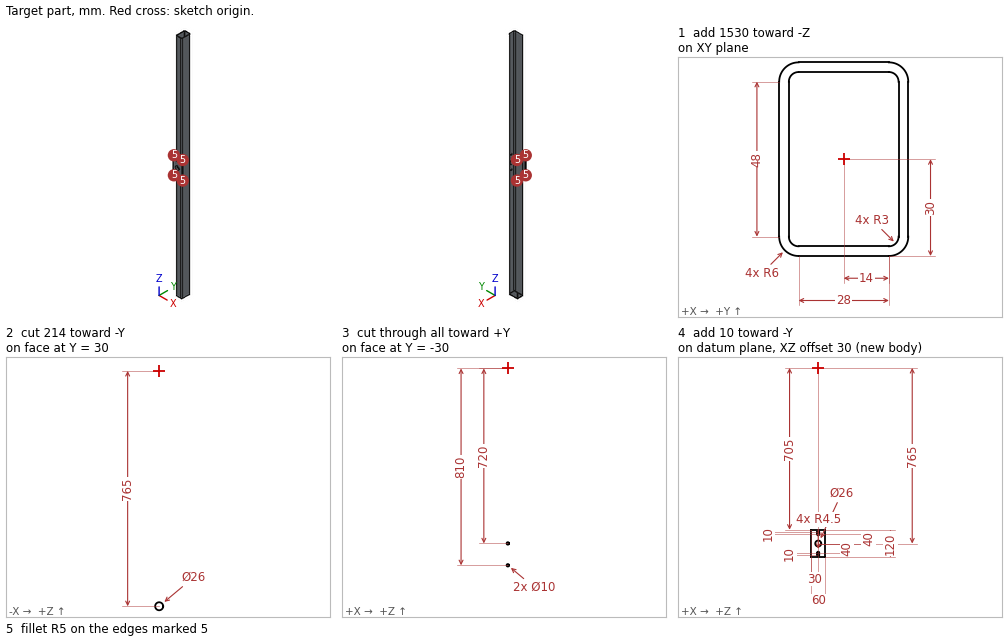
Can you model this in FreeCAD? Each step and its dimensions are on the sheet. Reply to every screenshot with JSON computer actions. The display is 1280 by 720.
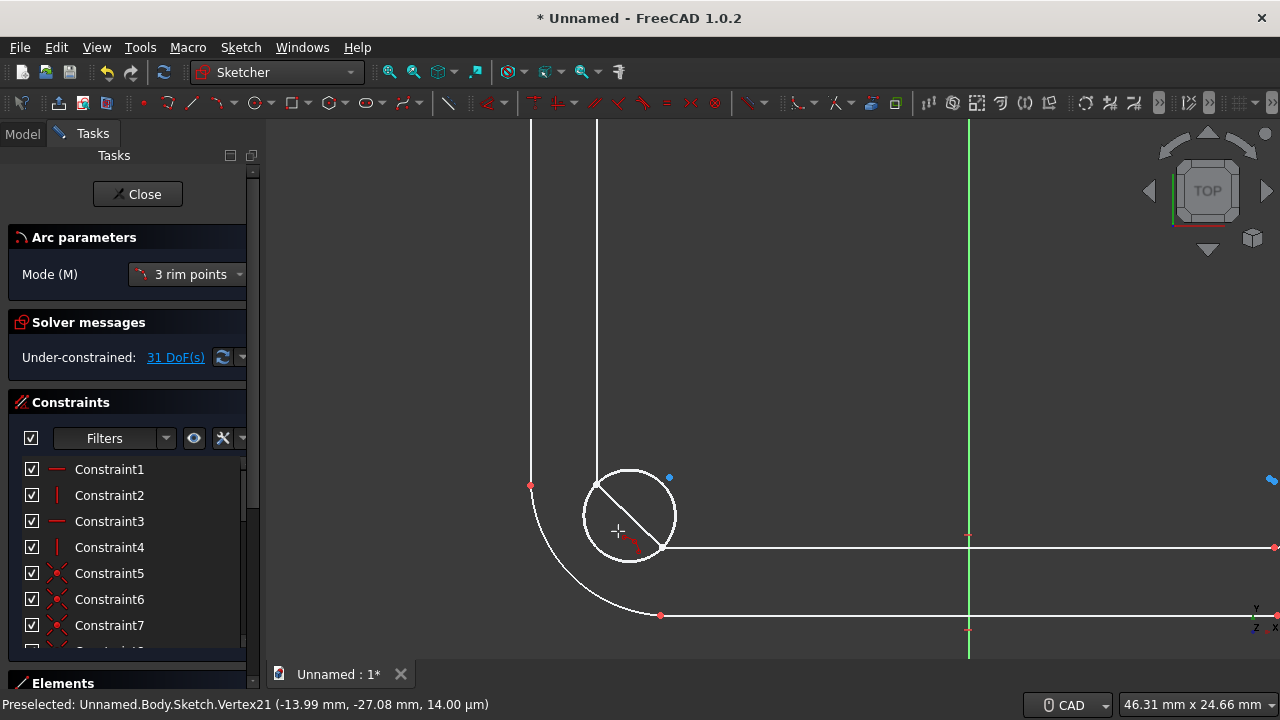
{"action": "left_click", "coordinate": [616, 527]}
{"action": "key", "text": "Escape"}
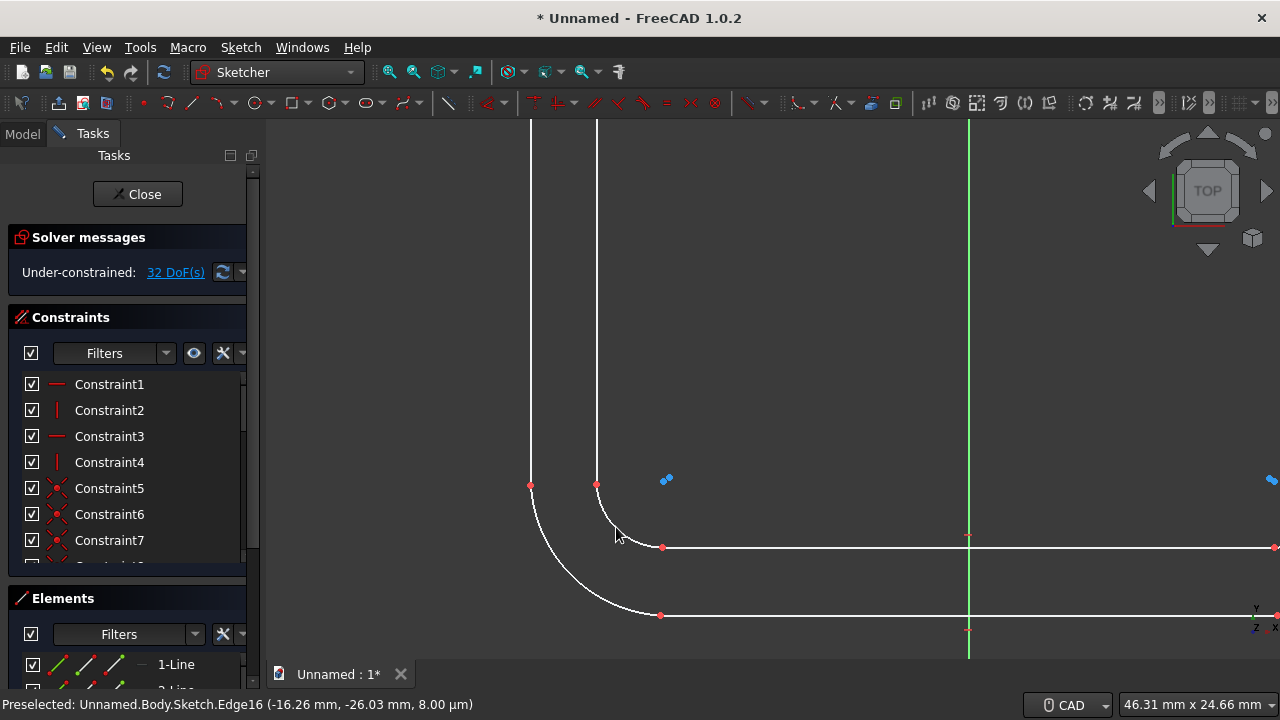
{"action": "scroll", "coordinate": [618, 531], "scroll_direction": "down", "scroll_amount": 7}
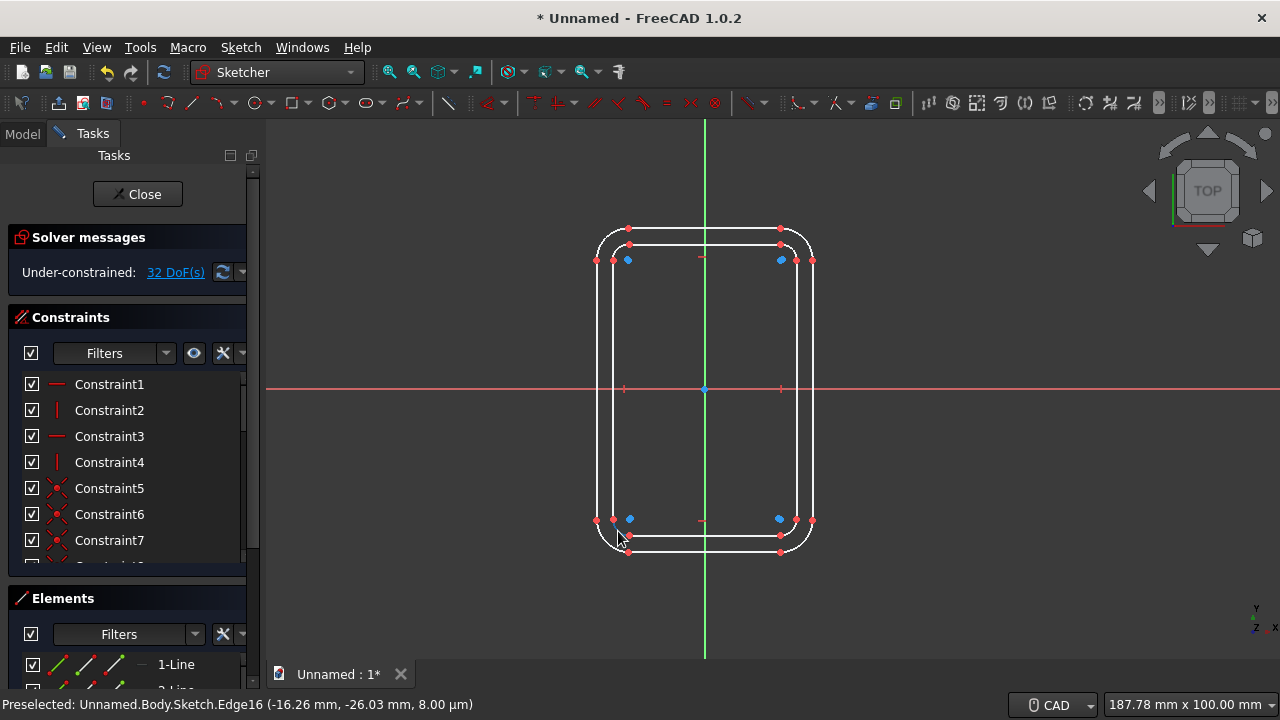
{"action": "left_click", "coordinate": [735, 552]}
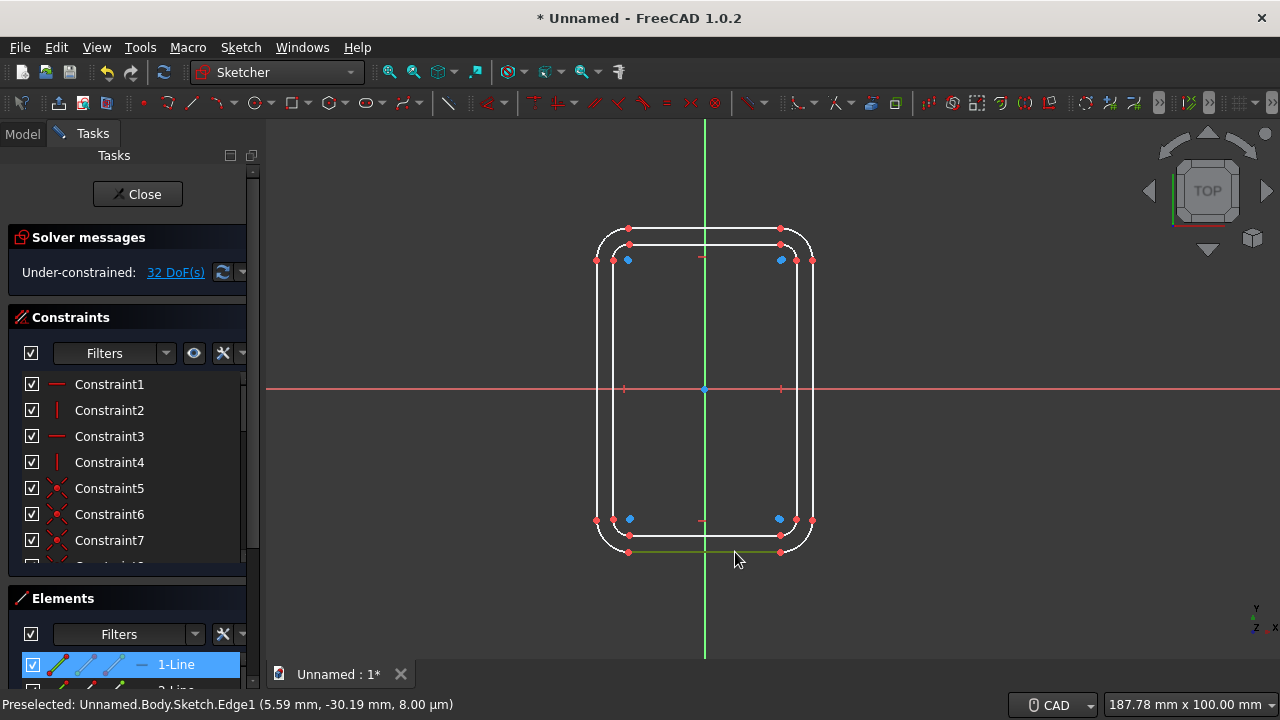
{"action": "left_click", "coordinate": [601, 535]}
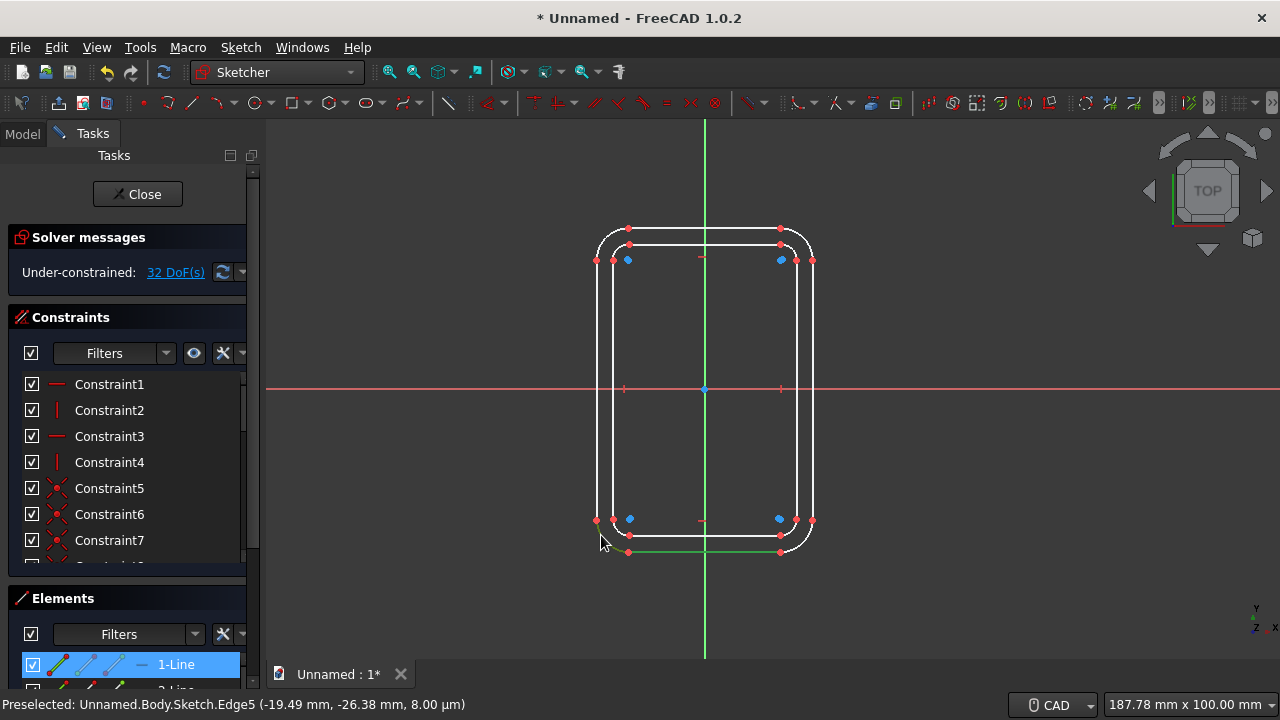
{"action": "left_click", "coordinate": [644, 104]}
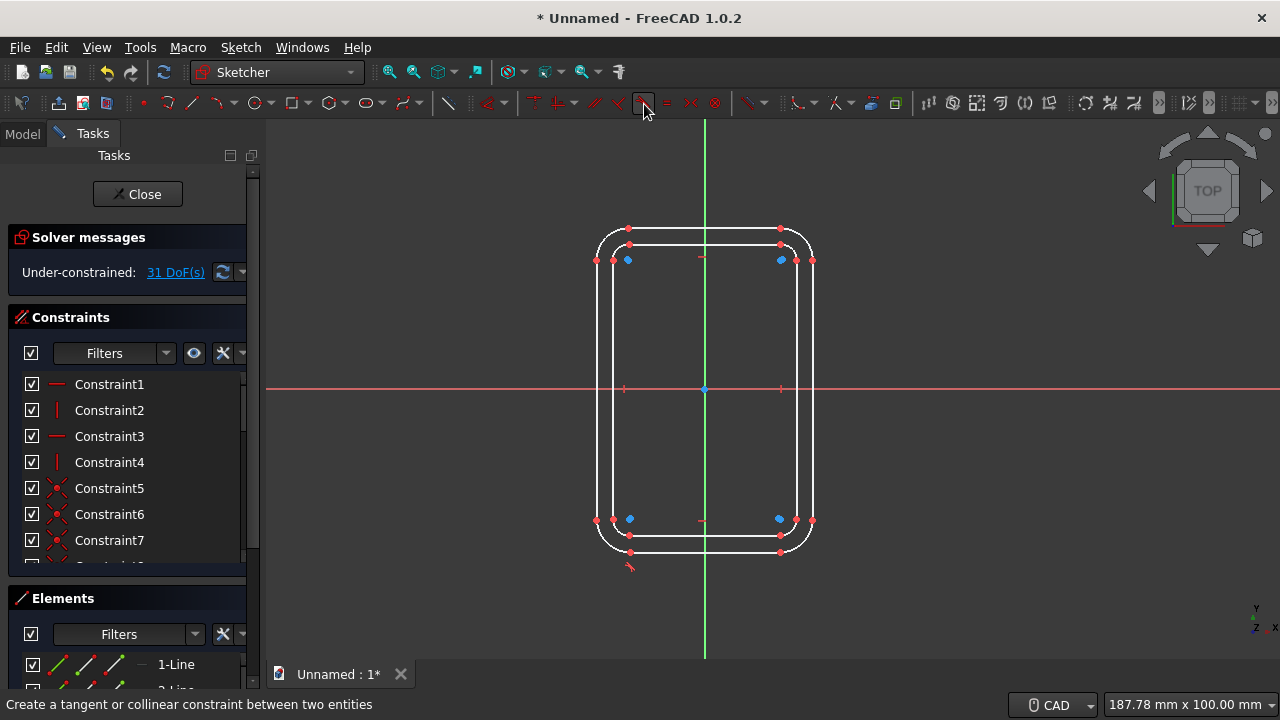
{"action": "left_click", "coordinate": [736, 553]}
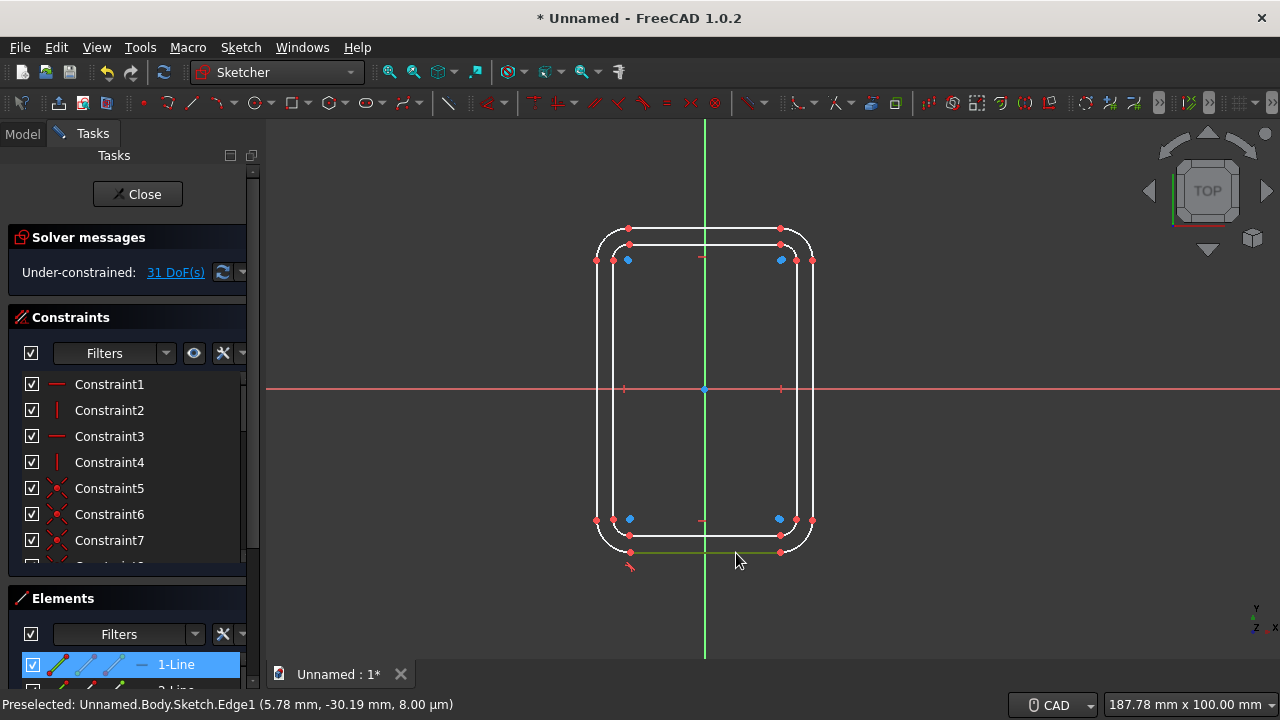
{"action": "left_click", "coordinate": [795, 549]}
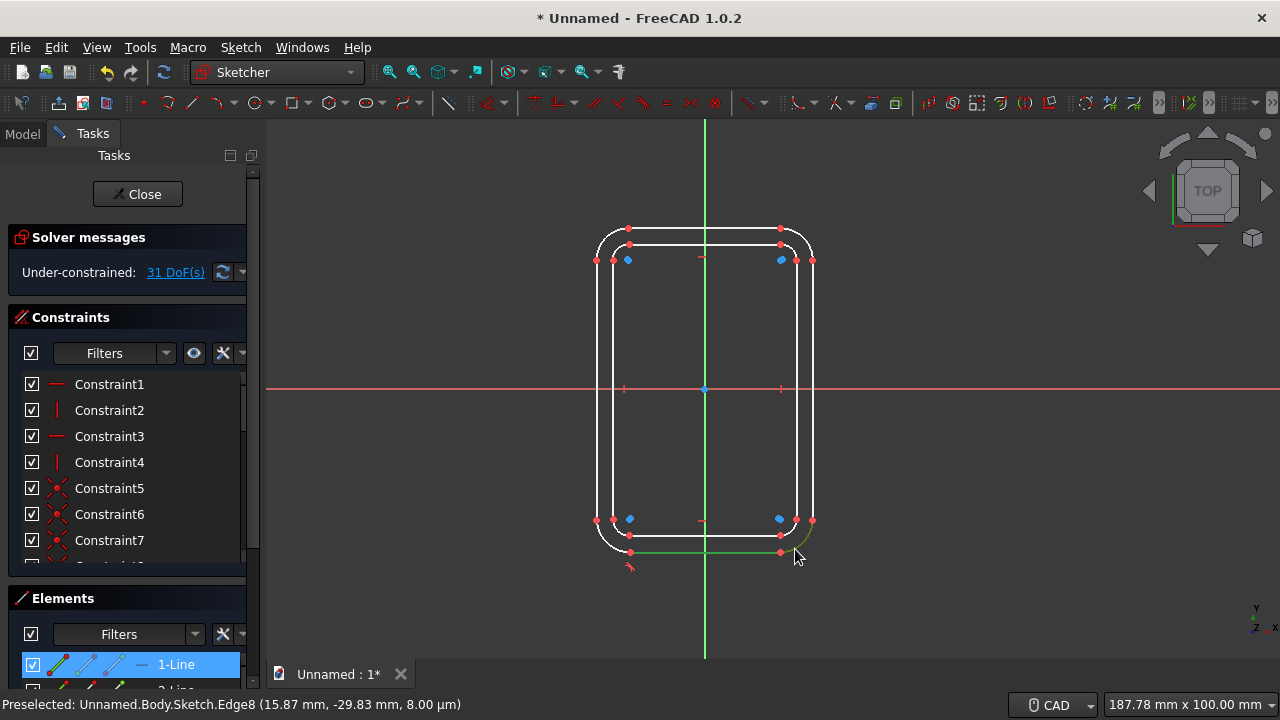
{"action": "left_click", "coordinate": [644, 104]}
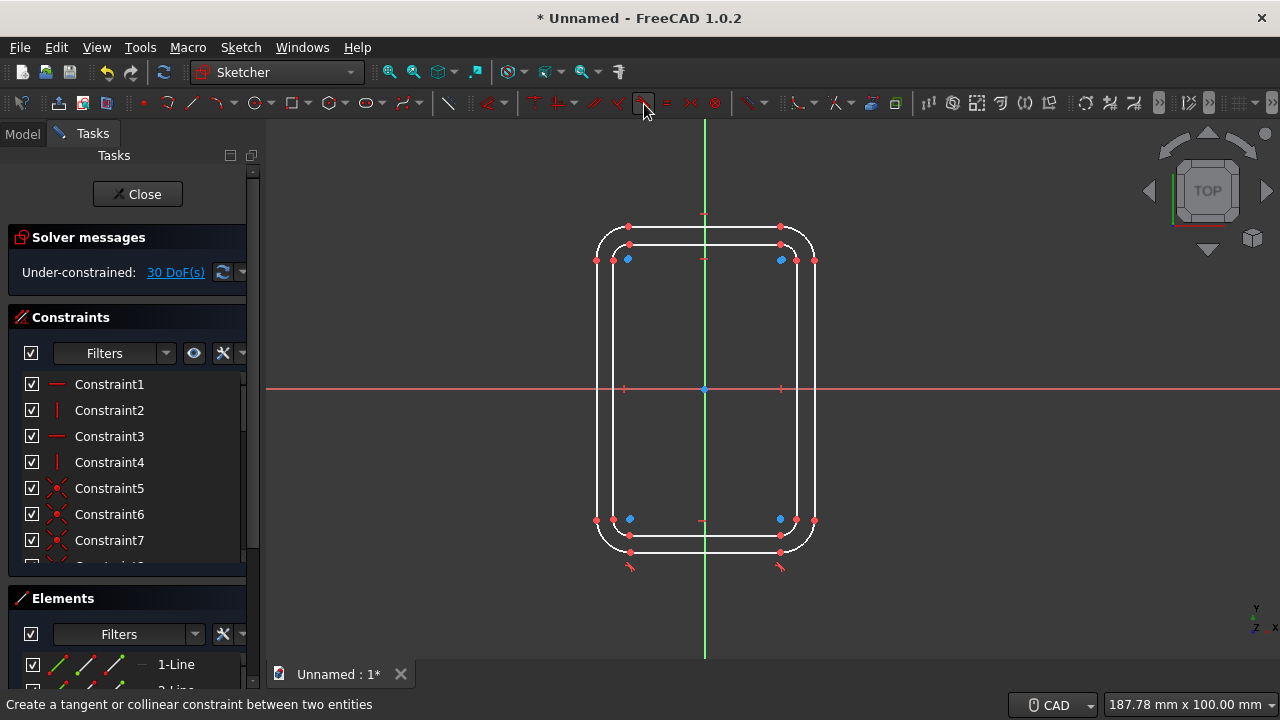
{"action": "left_click", "coordinate": [597, 442]}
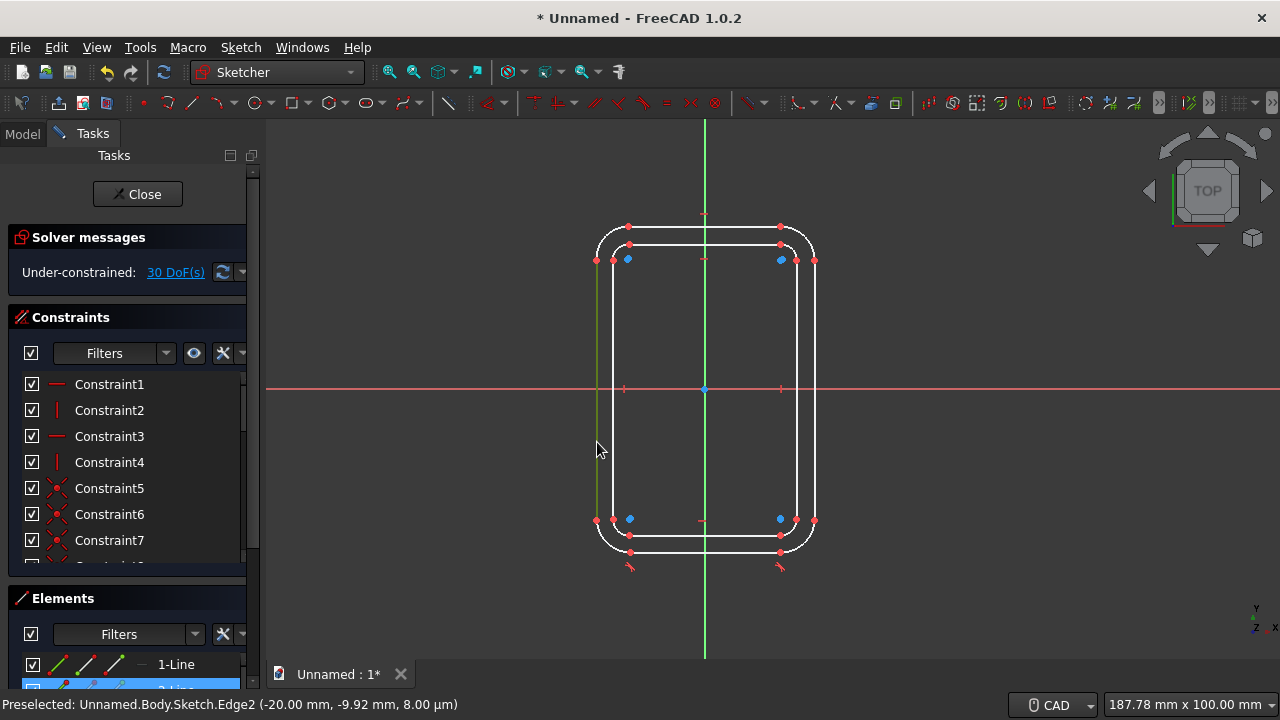
{"action": "left_click", "coordinate": [601, 535]}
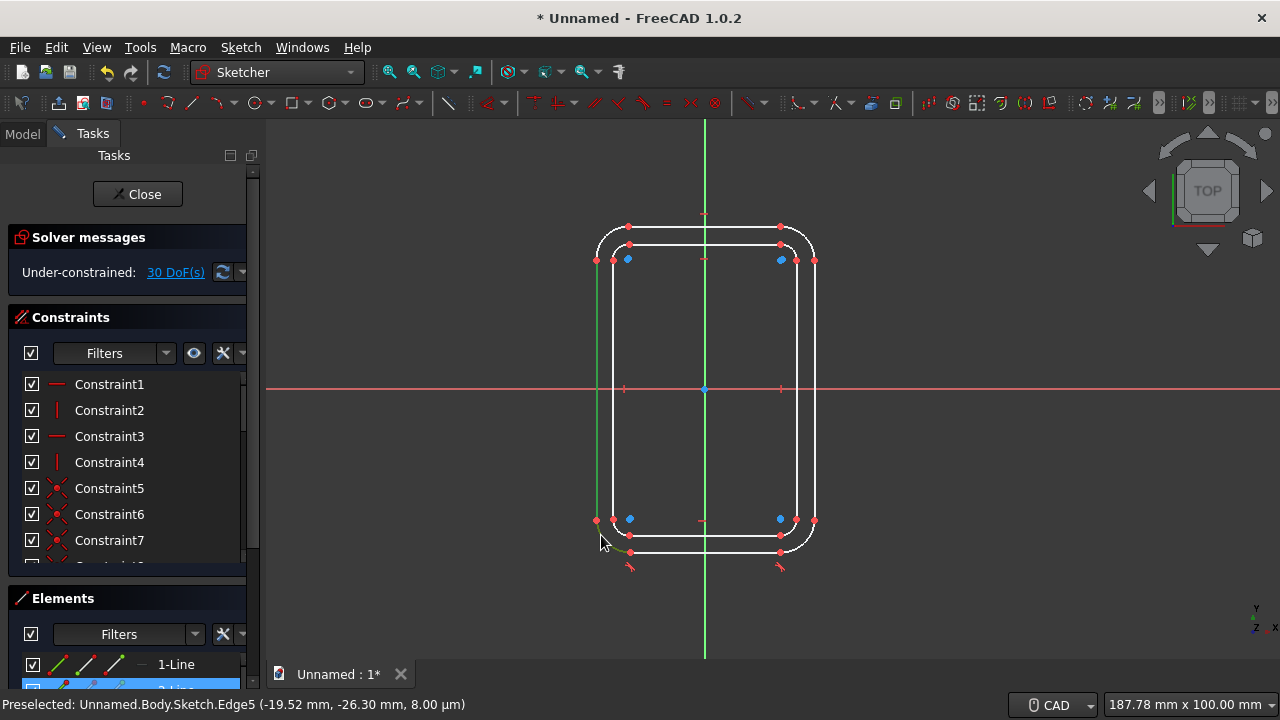
{"action": "left_click", "coordinate": [644, 104]}